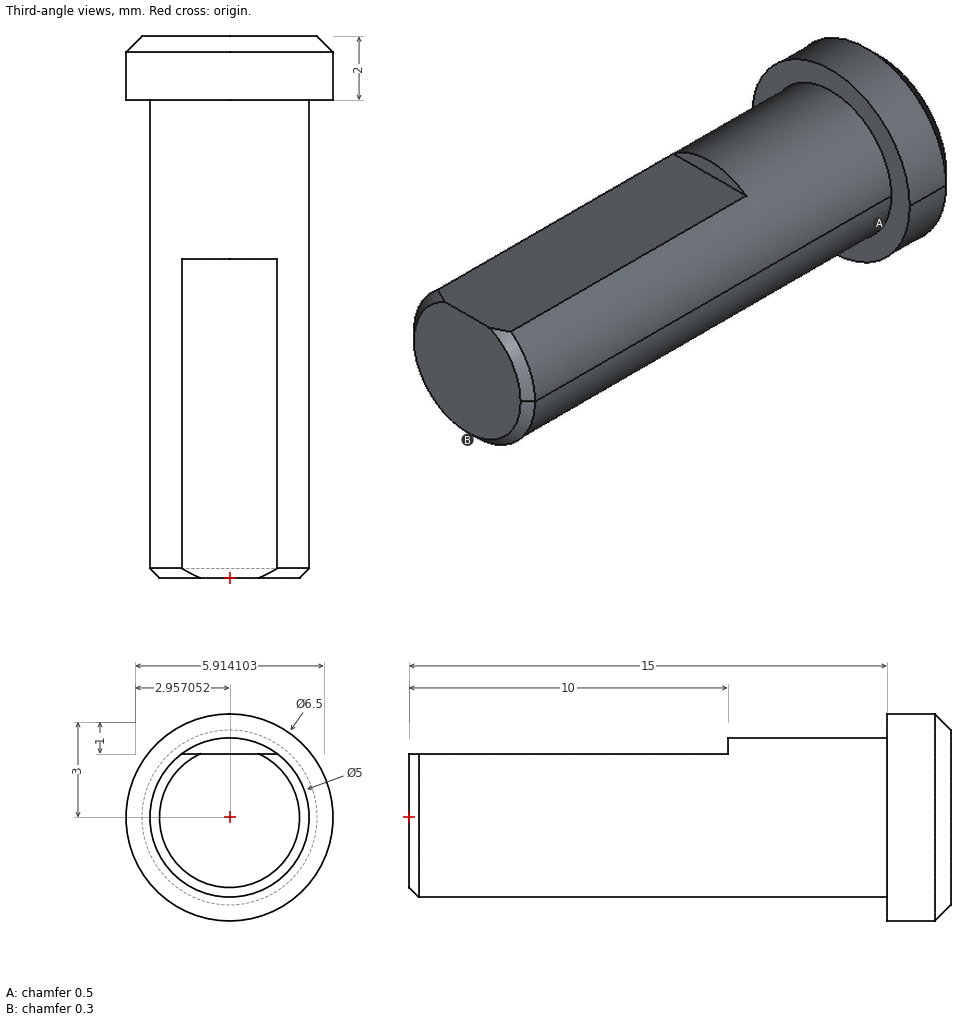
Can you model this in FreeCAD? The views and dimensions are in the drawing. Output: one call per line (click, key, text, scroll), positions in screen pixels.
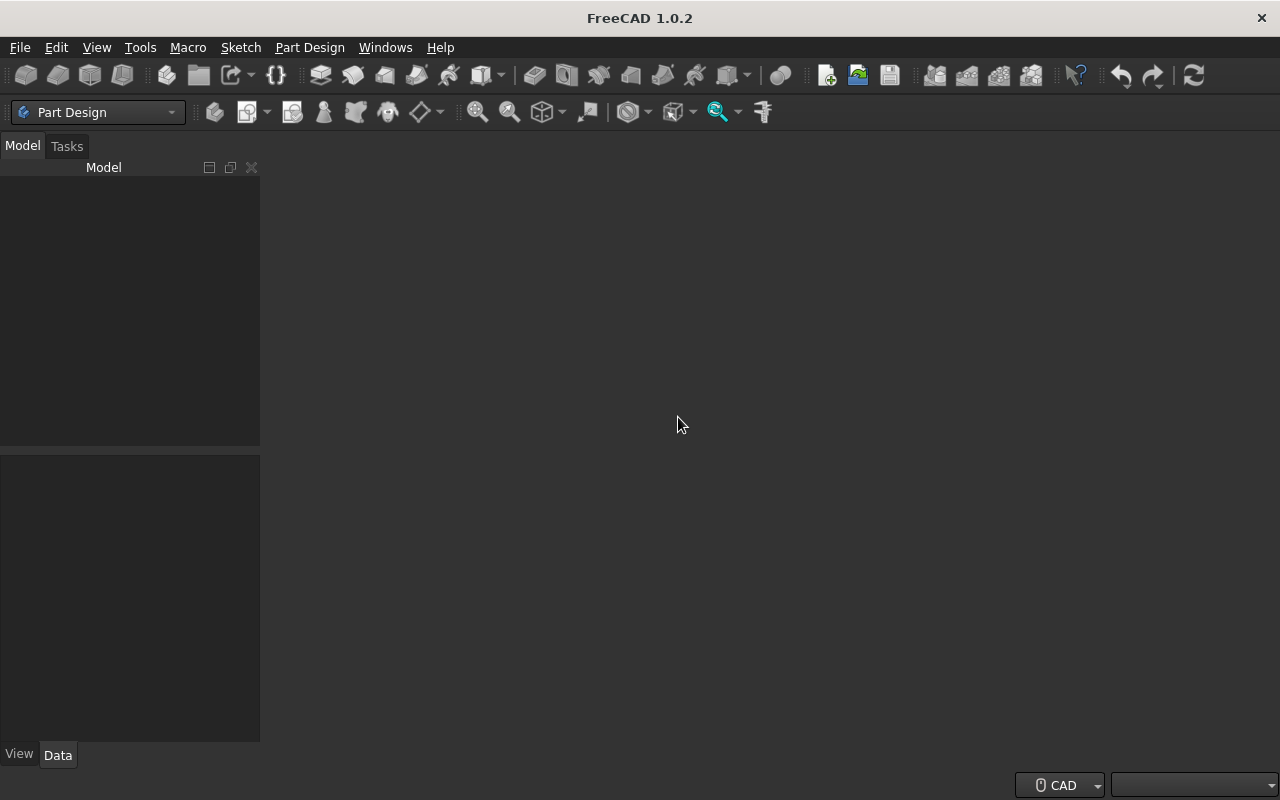
click(826, 76)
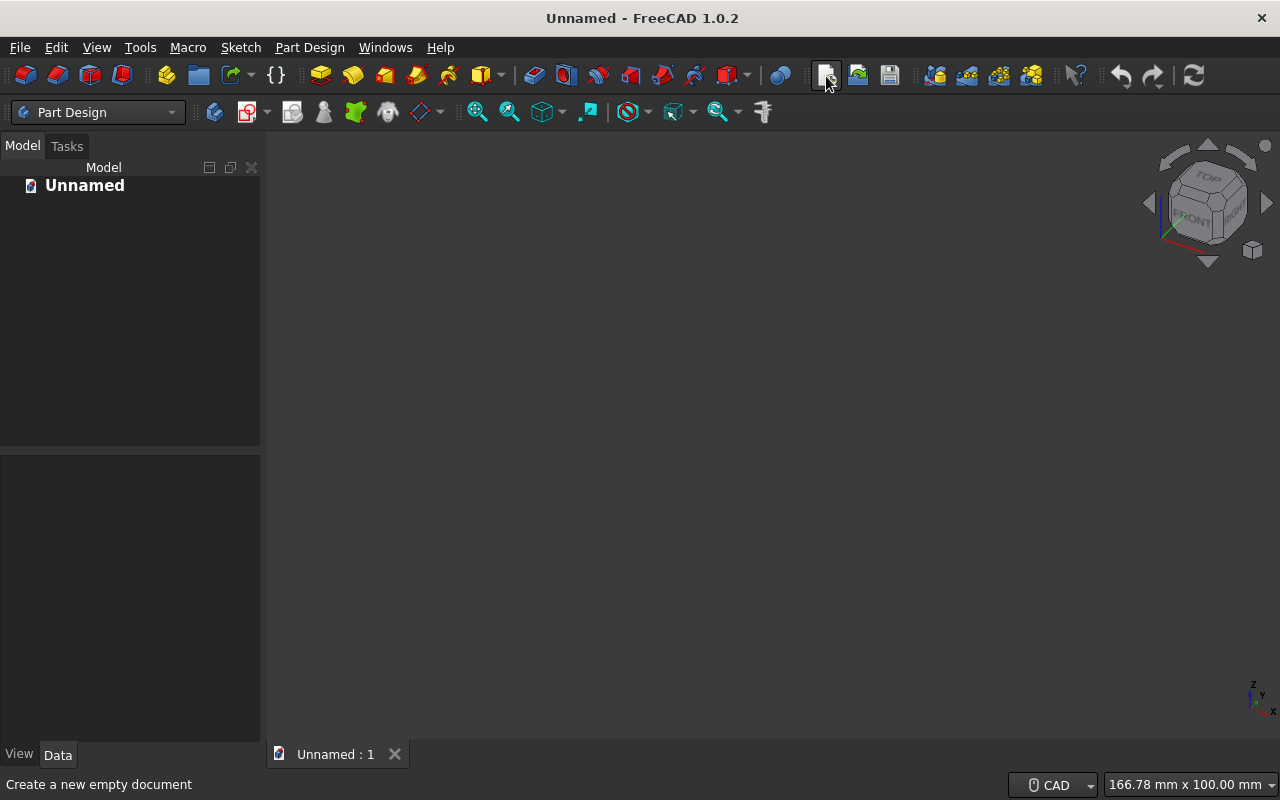
click(248, 112)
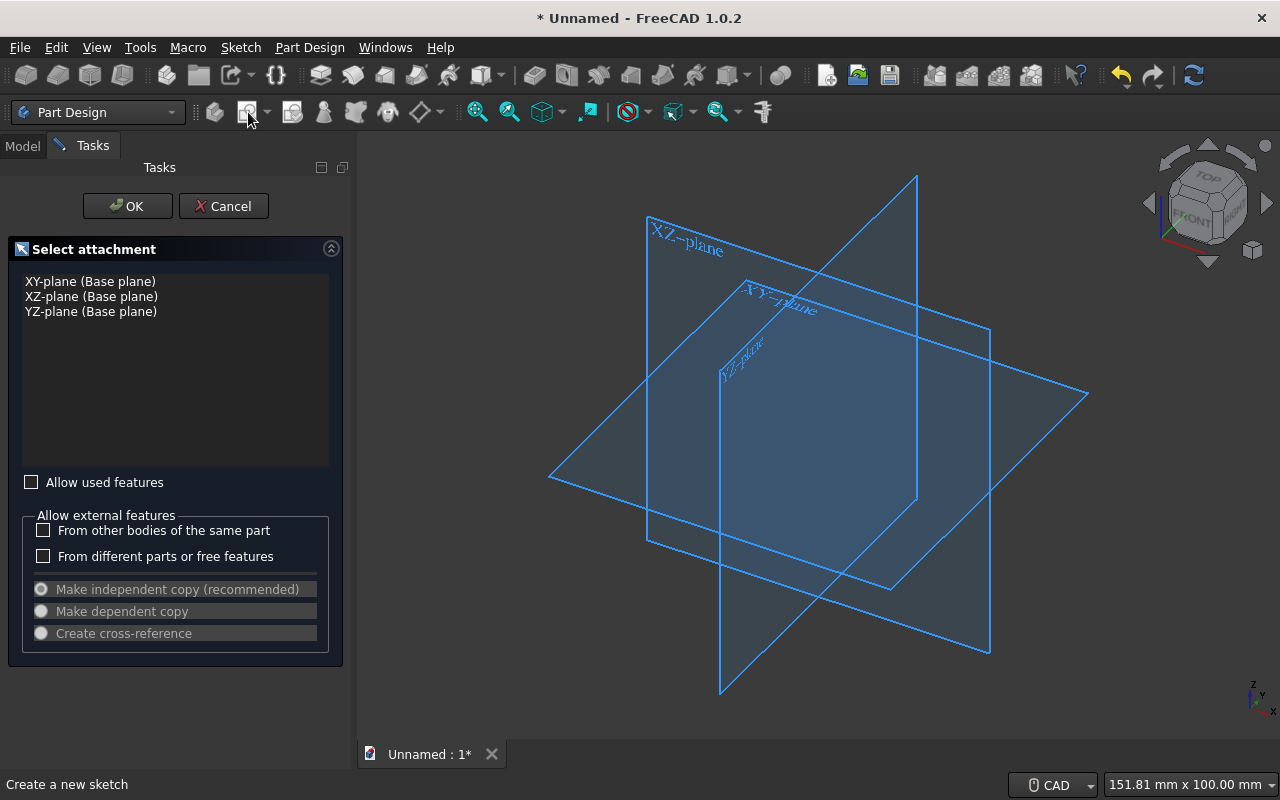
click(82, 296)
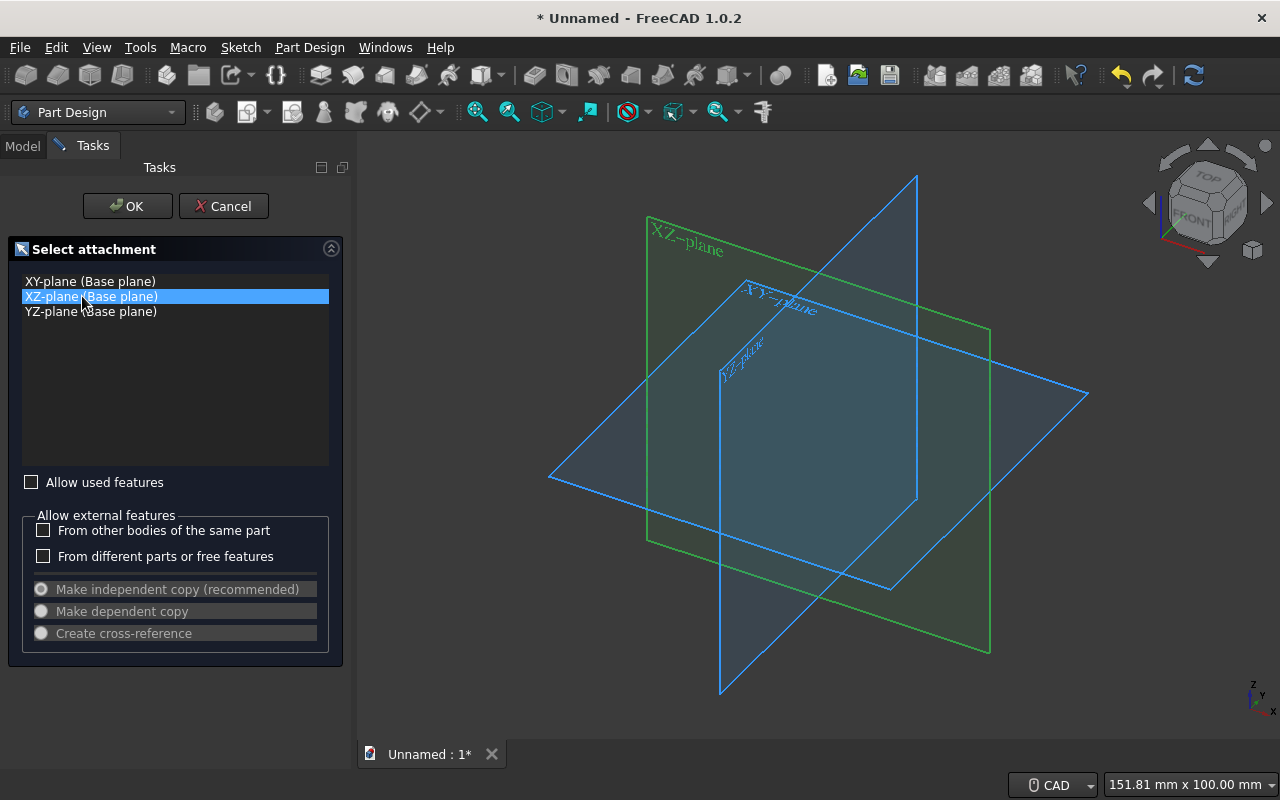
click(128, 206)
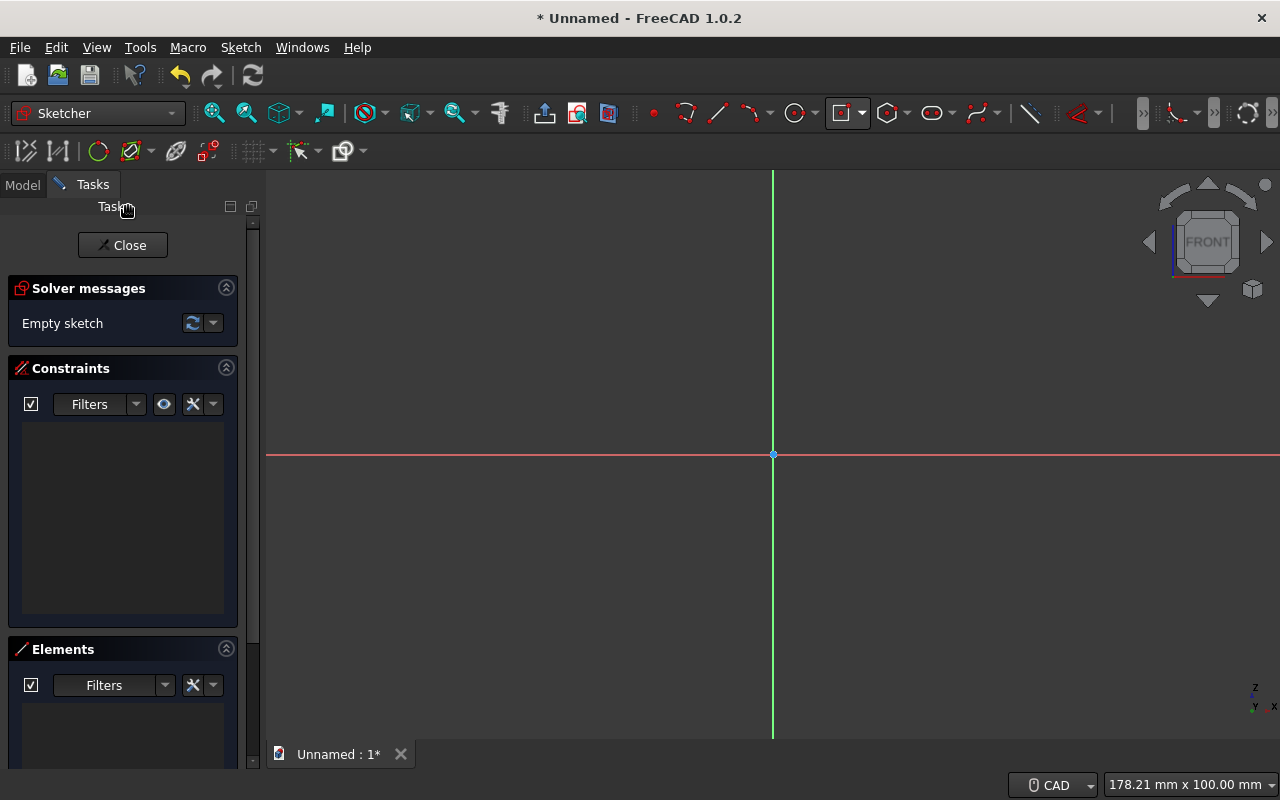
scroll(778, 454, up, 13)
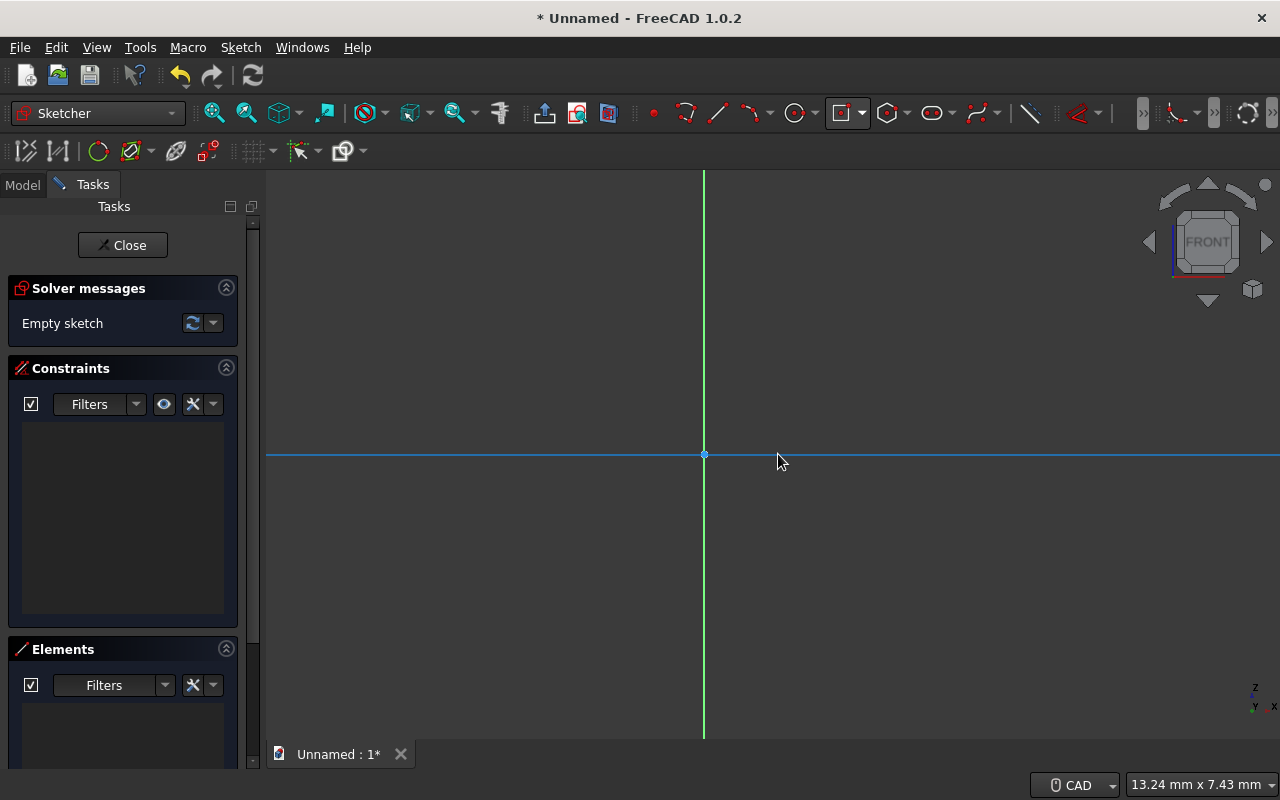
click(796, 114)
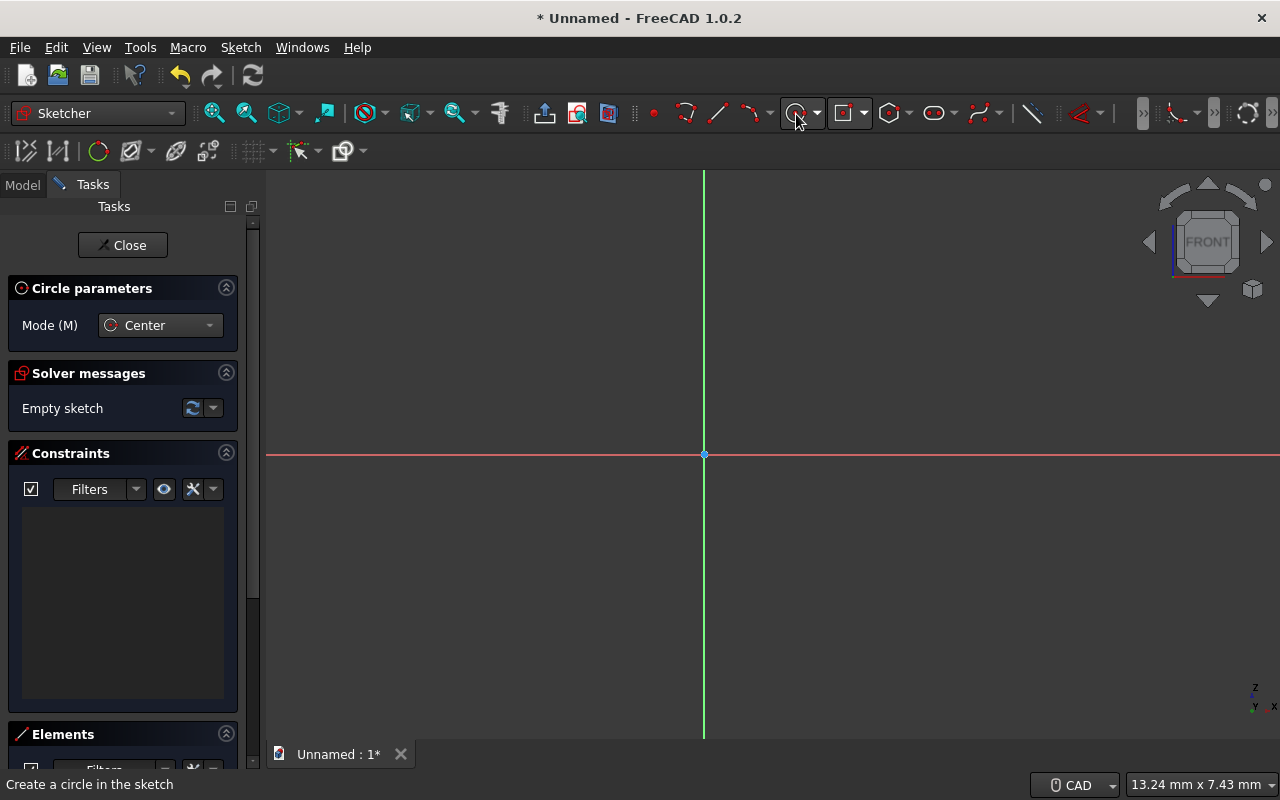
click(704, 454)
click(840, 319)
key(Escape)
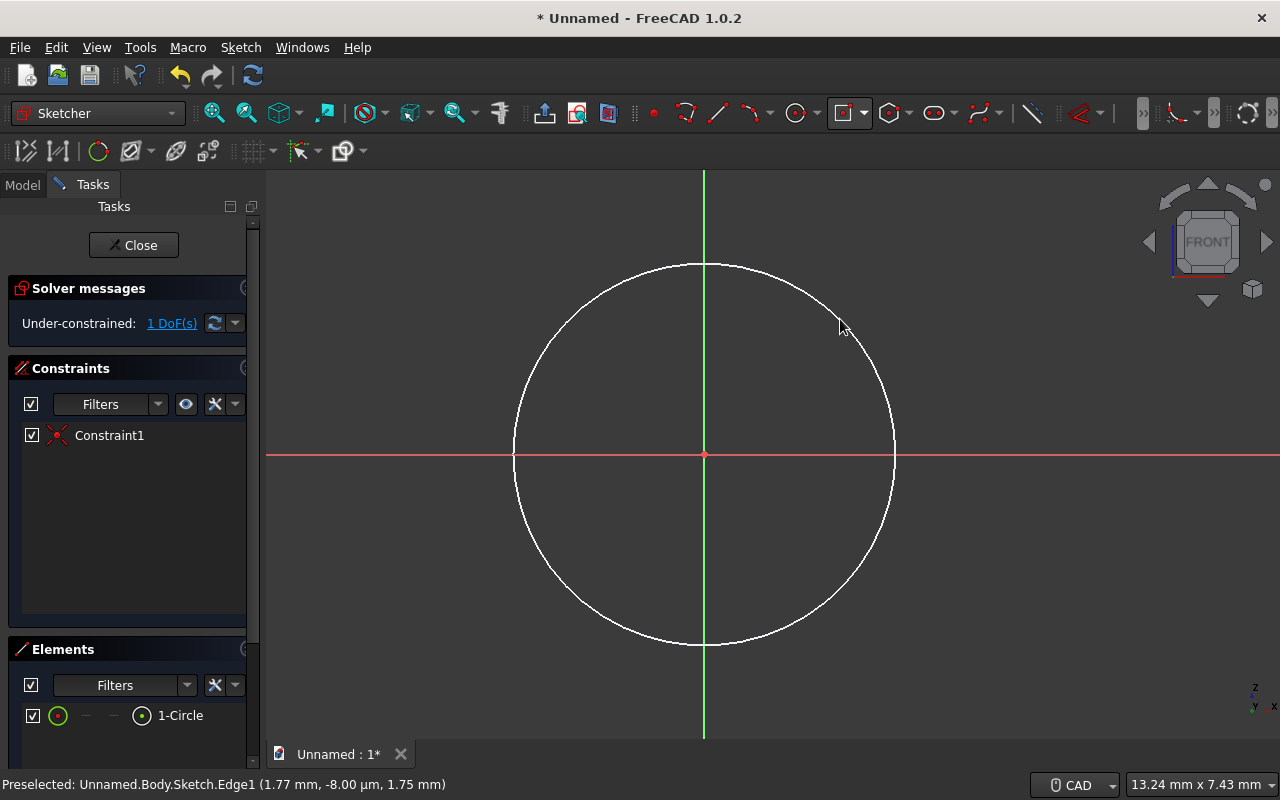
click(1080, 114)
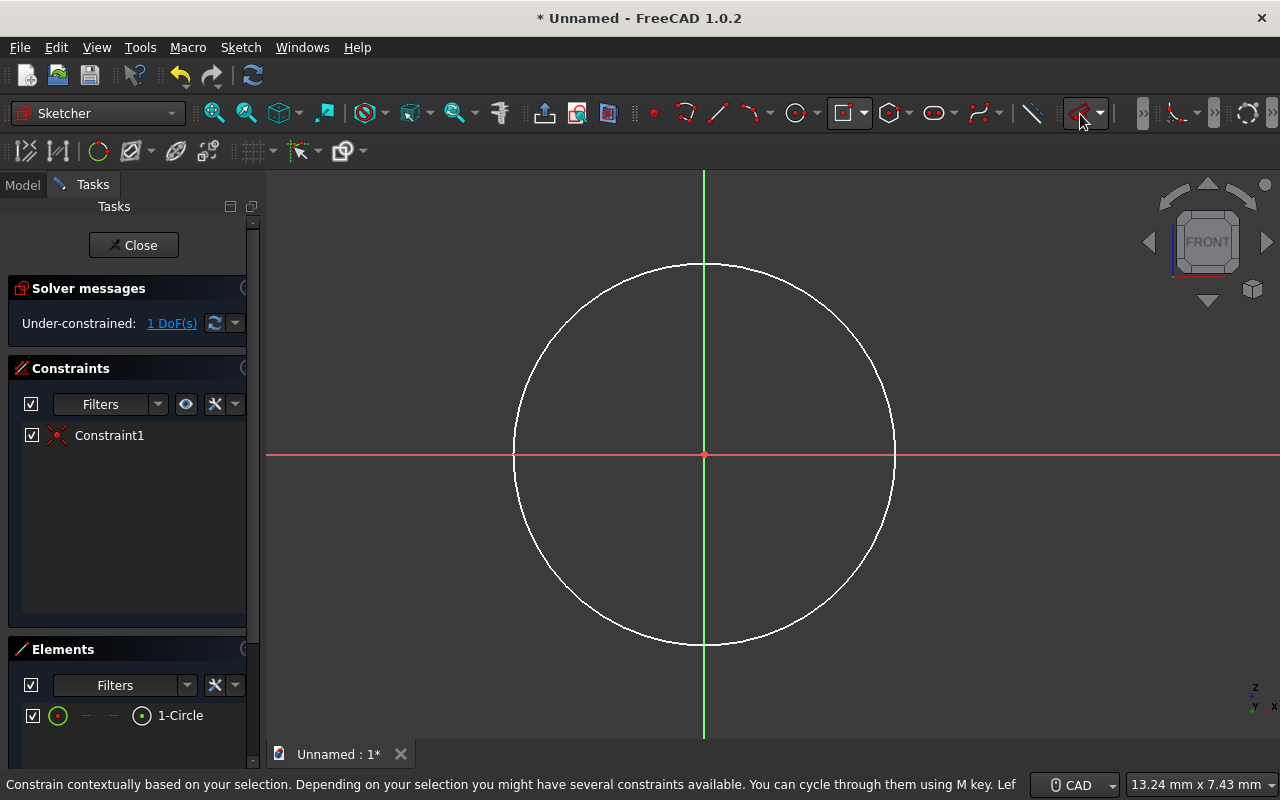
click(839, 319)
click(862, 296)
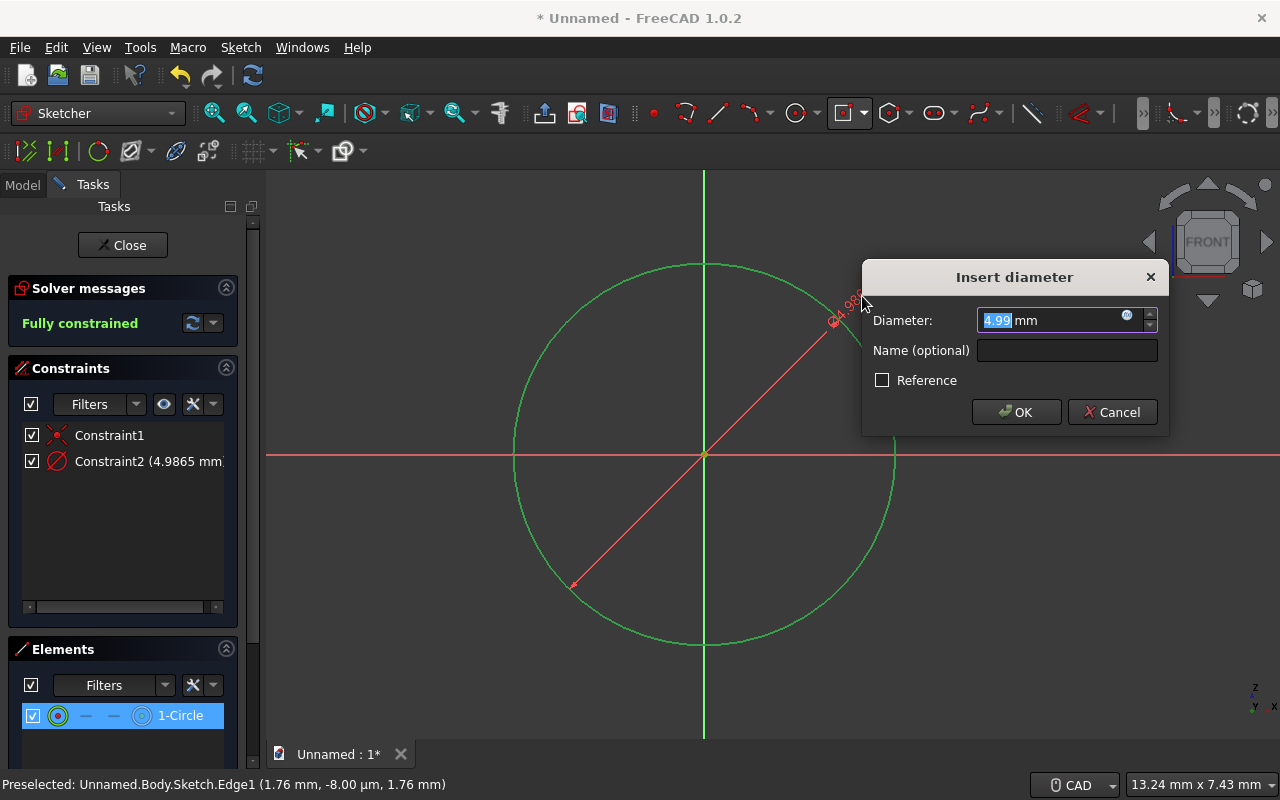
text(5)
key(Return)
key(Escape)